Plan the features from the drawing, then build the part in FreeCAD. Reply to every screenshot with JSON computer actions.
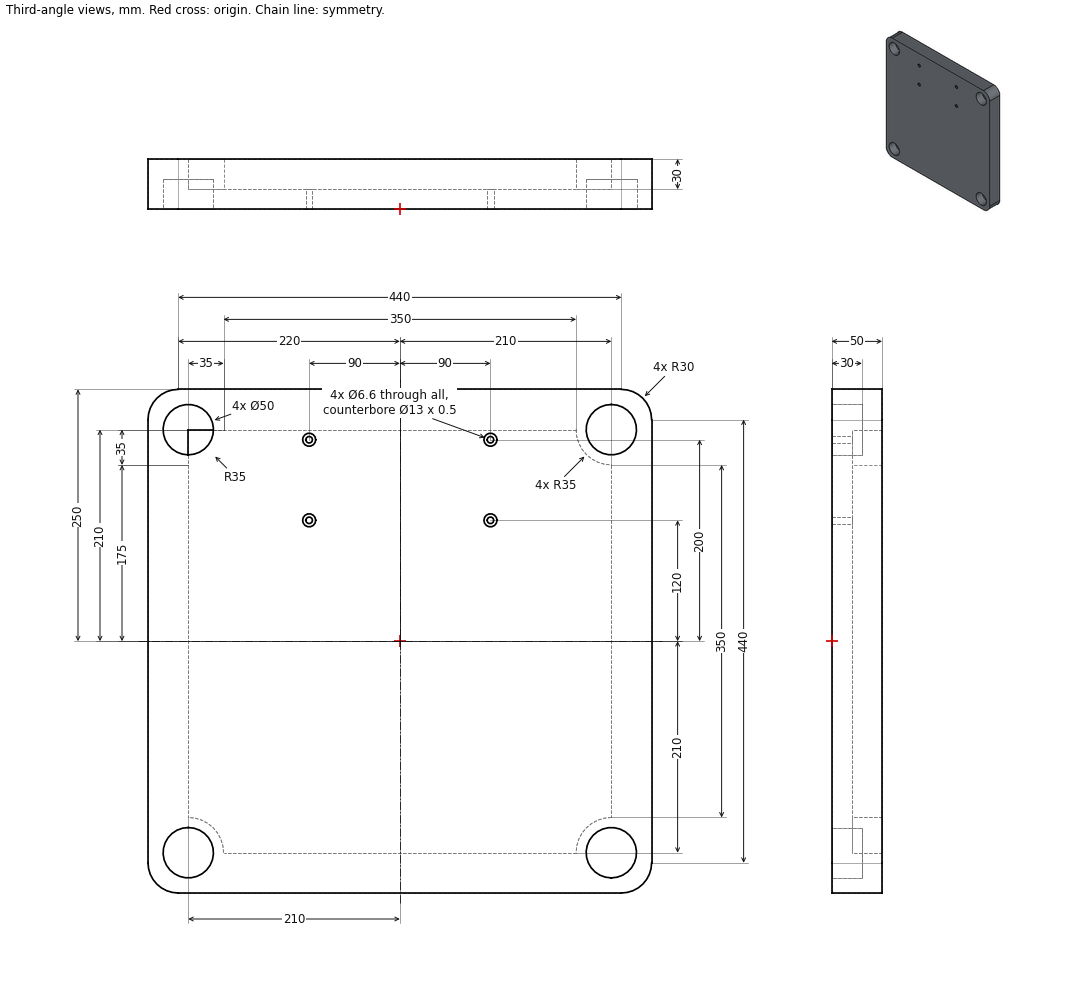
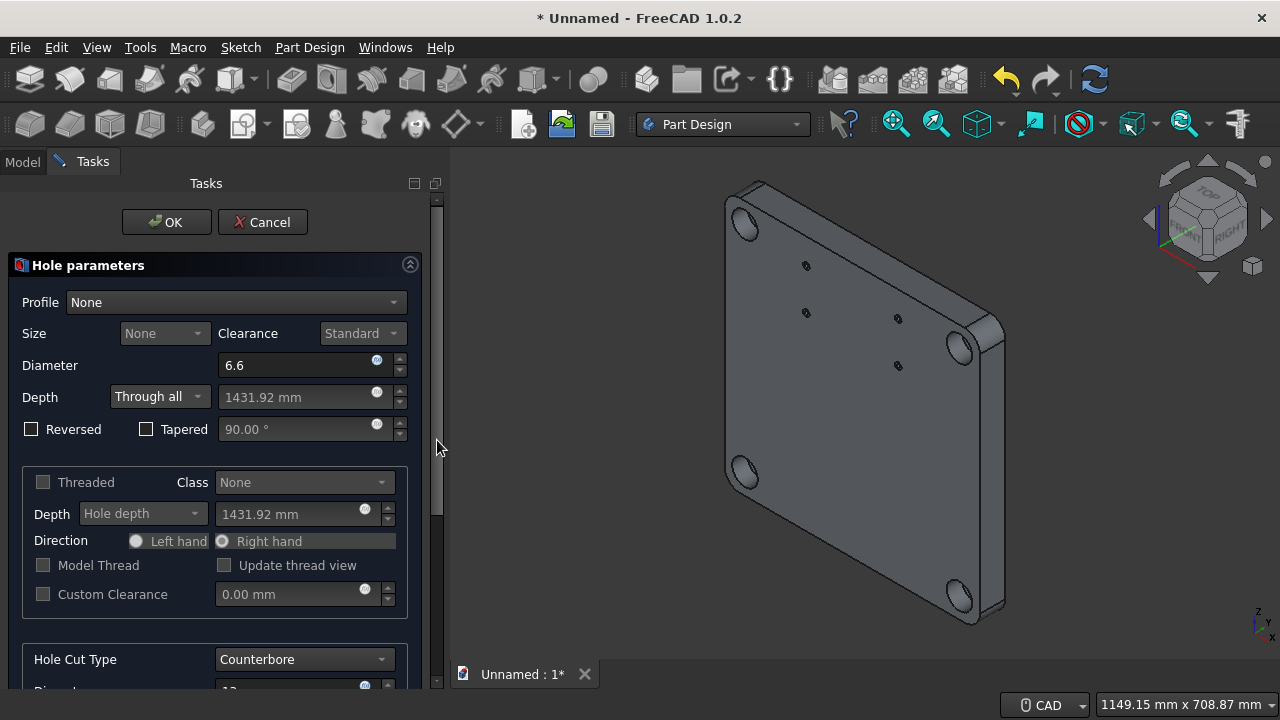
{"action": "left_click", "coordinate": [167, 222]}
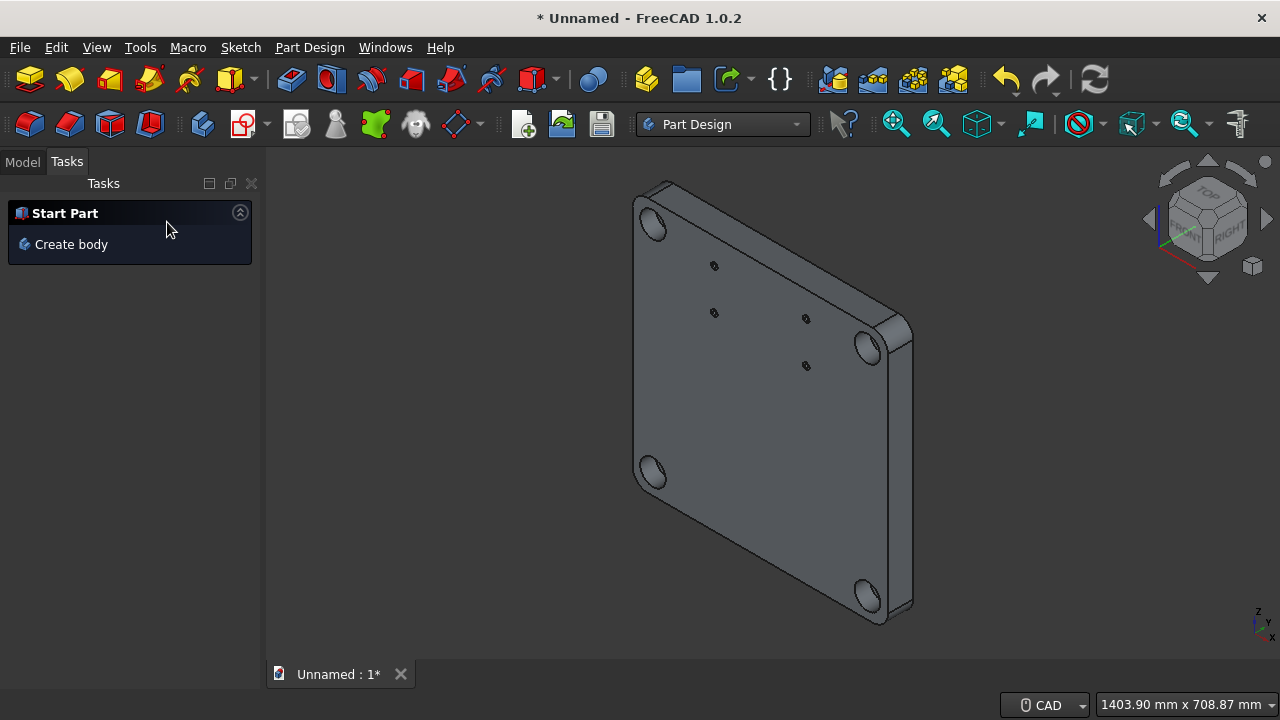
{"action": "key", "text": "4"}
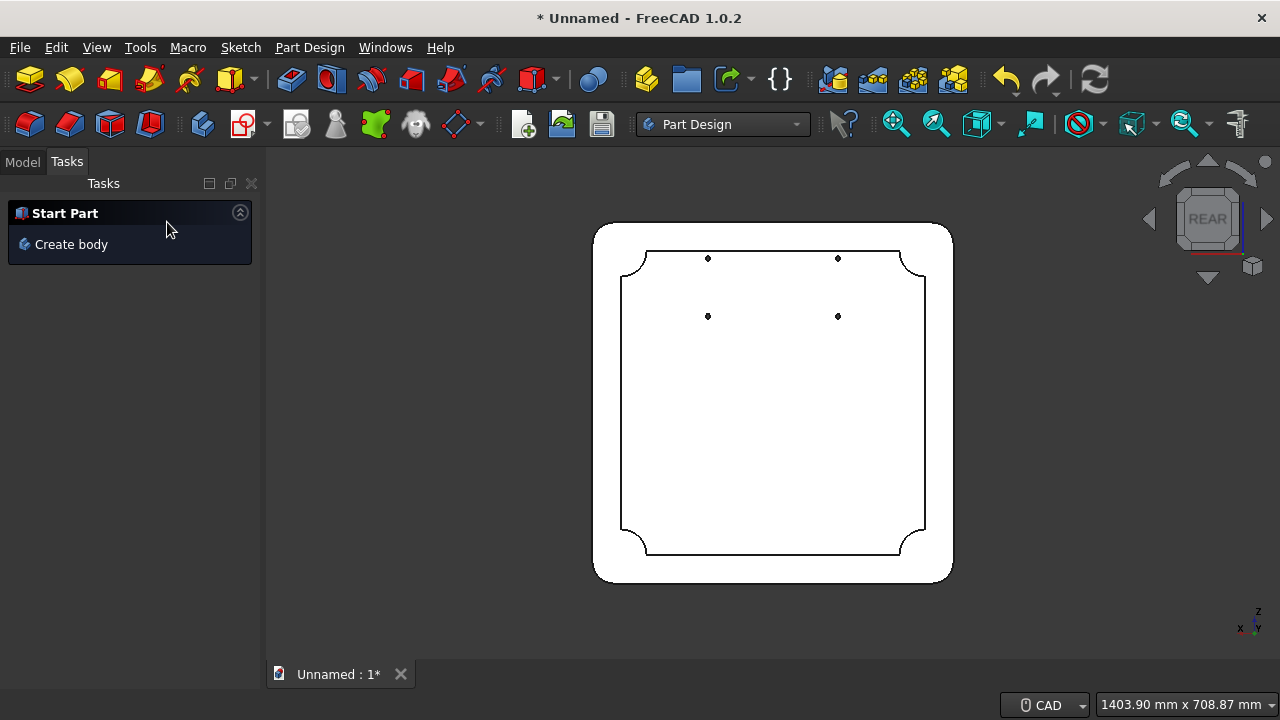
{"action": "left_click", "coordinate": [618, 247]}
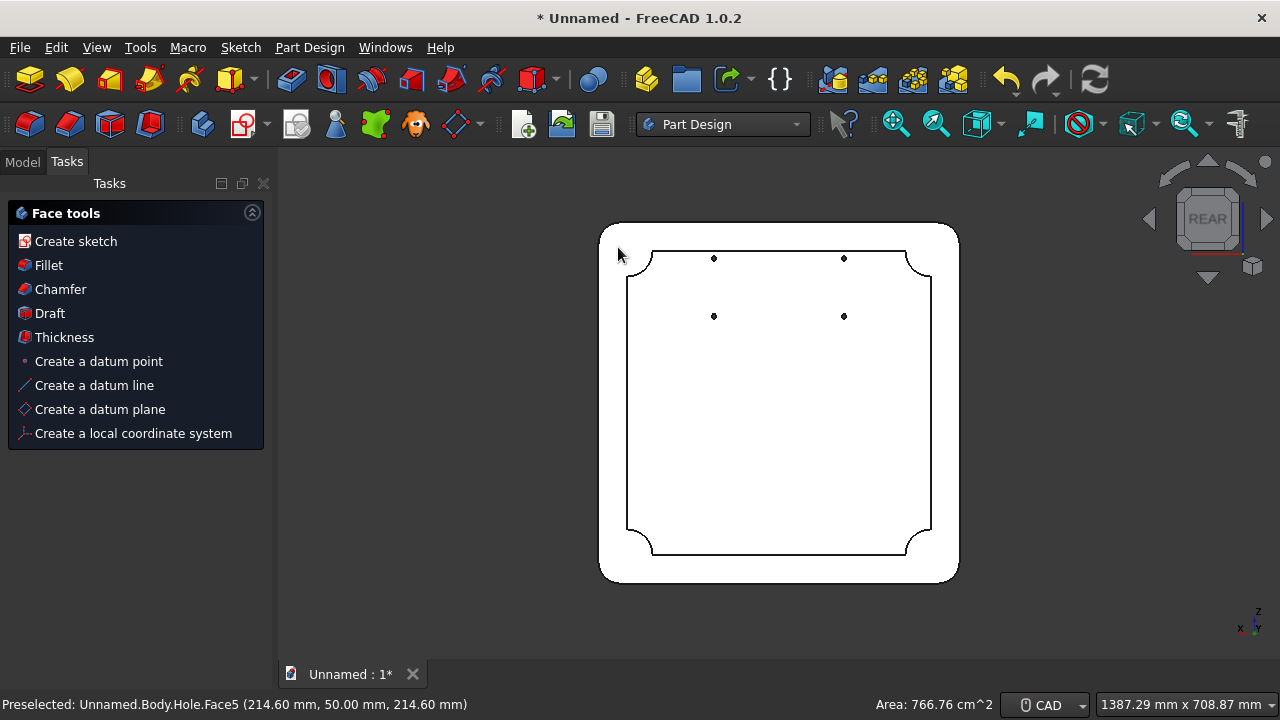
{"action": "left_click", "coordinate": [244, 124]}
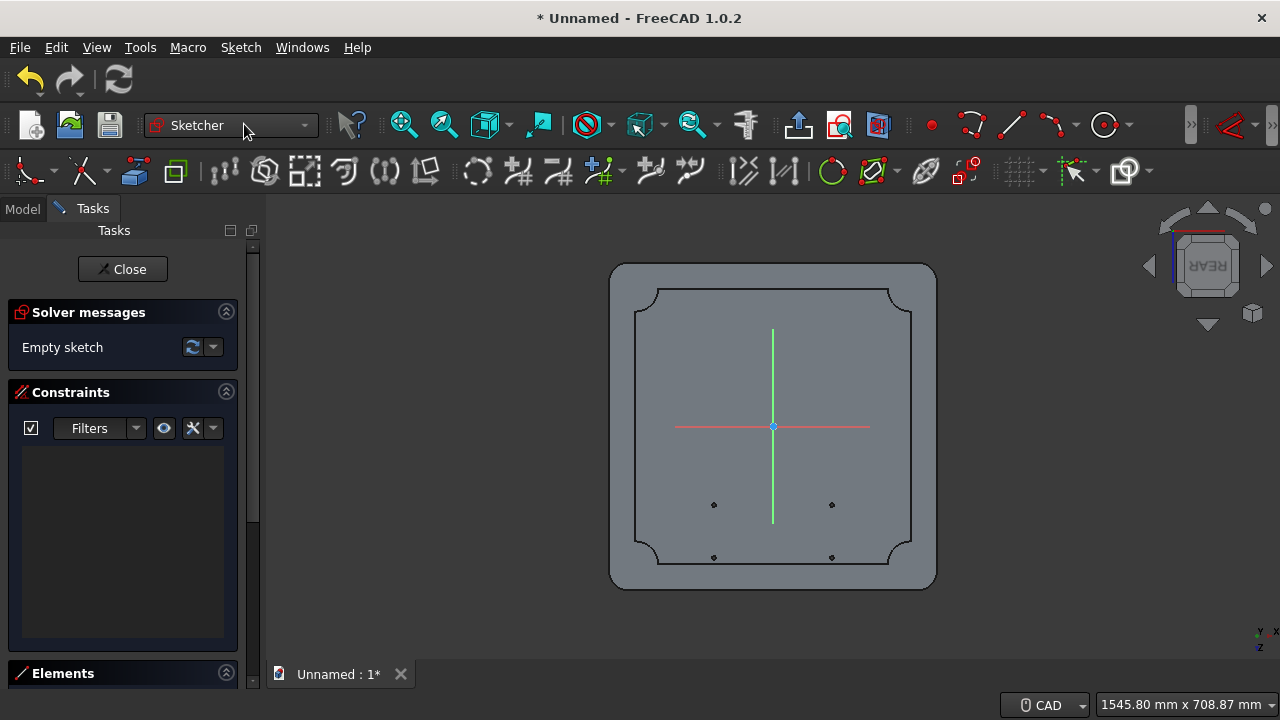
{"action": "scroll", "coordinate": [642, 563], "scroll_direction": "up", "scroll_amount": 13}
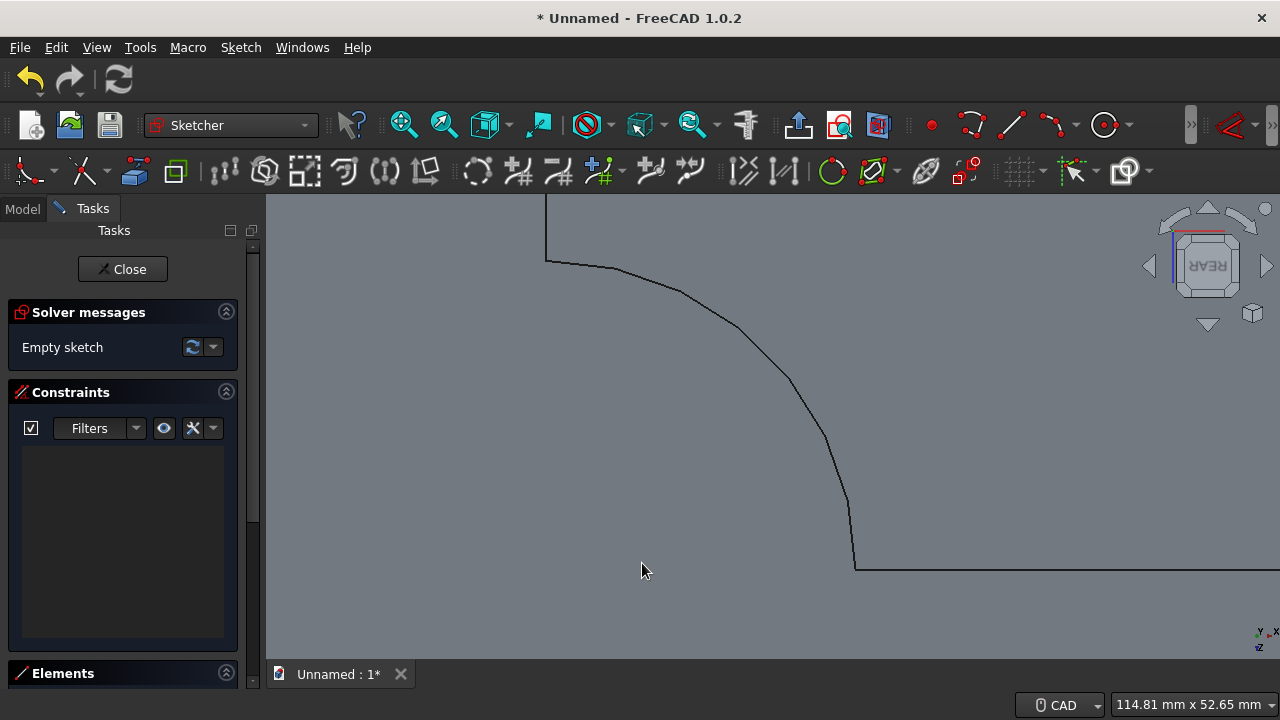
{"action": "left_click", "coordinate": [972, 126]}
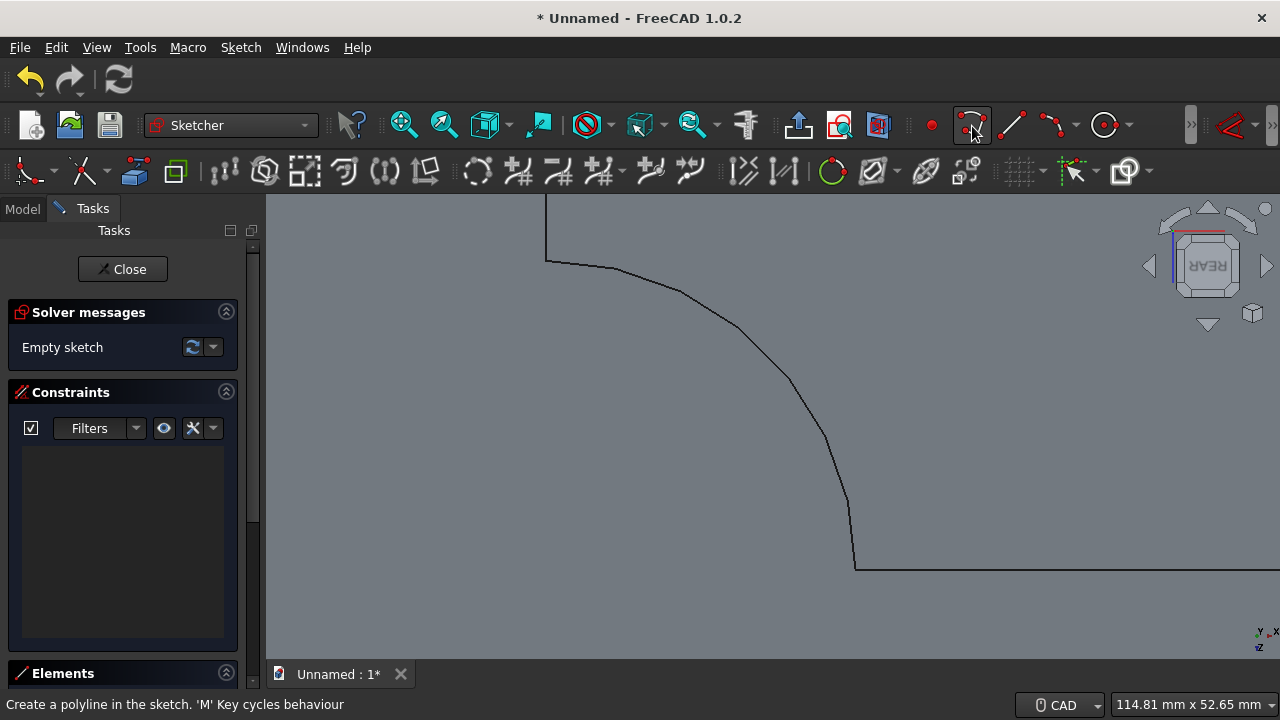
{"action": "left_click", "coordinate": [546, 261]}
{"action": "left_click", "coordinate": [546, 570]}
{"action": "left_click", "coordinate": [856, 570]}
{"action": "right_click", "coordinate": [856, 570]}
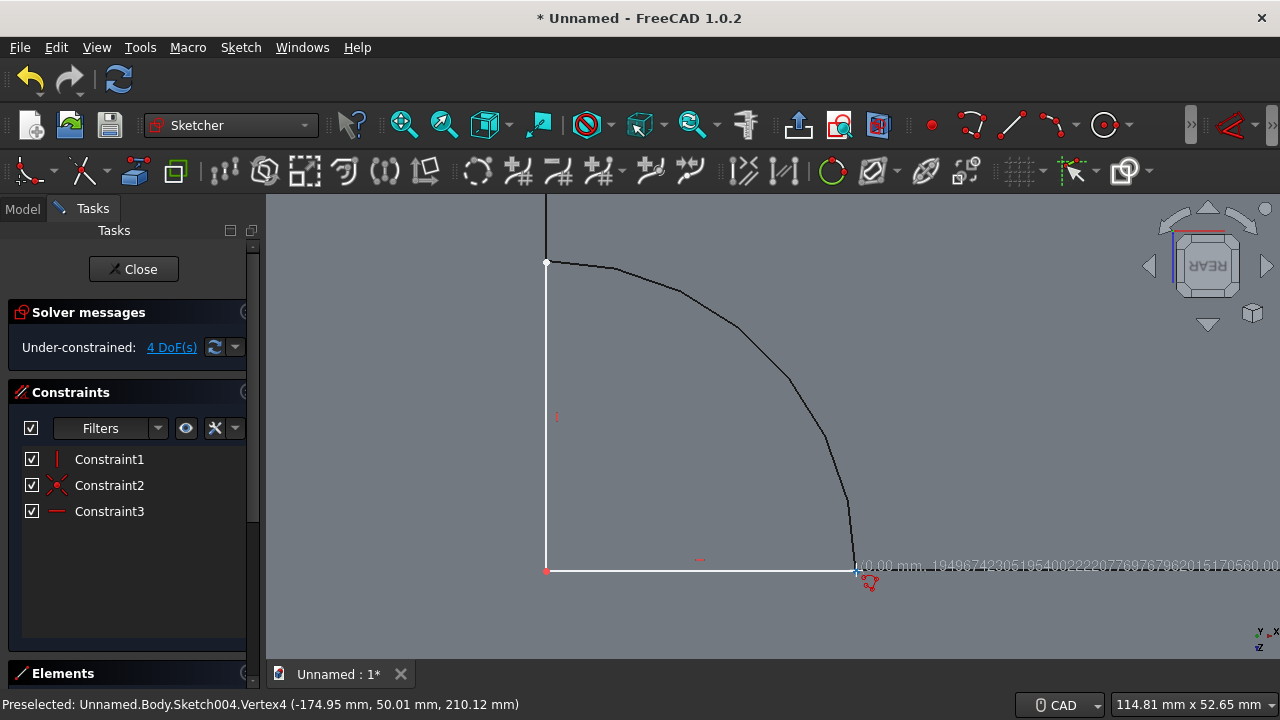
{"action": "key", "text": "g 3 a"}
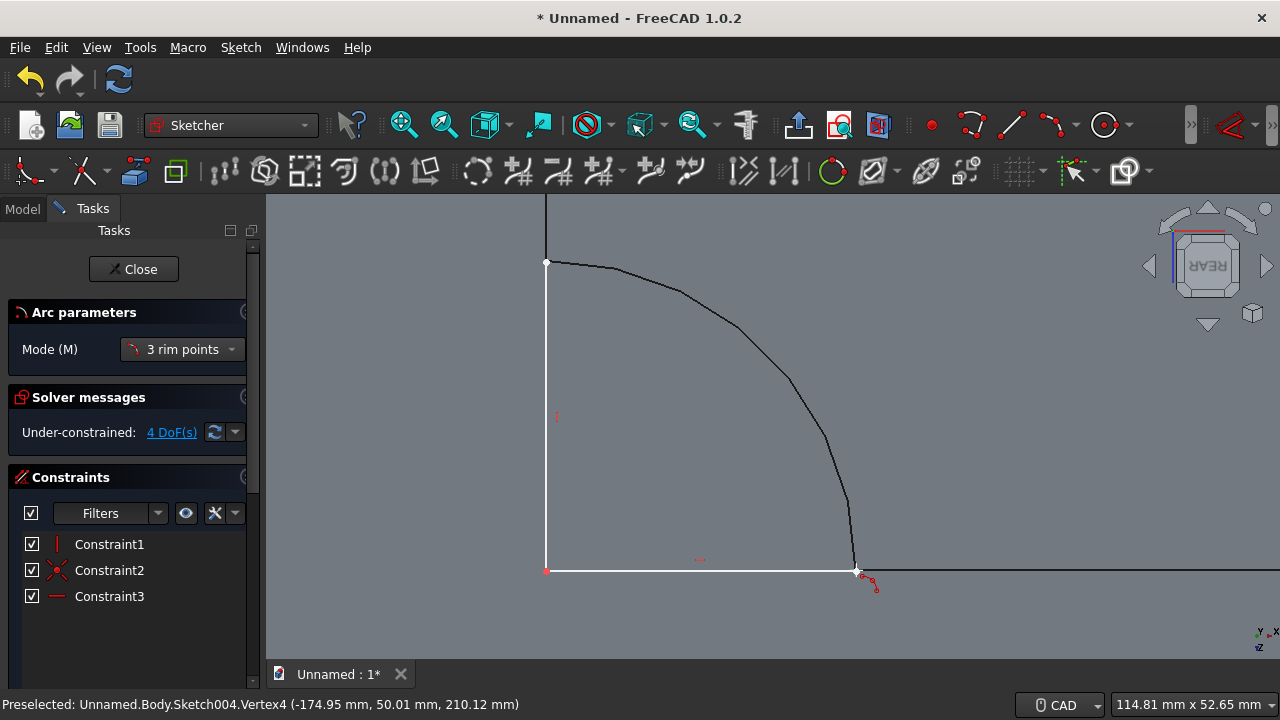
{"action": "left_click", "coordinate": [856, 571]}
{"action": "left_click", "coordinate": [546, 262]}
{"action": "left_click", "coordinate": [765, 351]}
{"action": "key", "text": "Escape"}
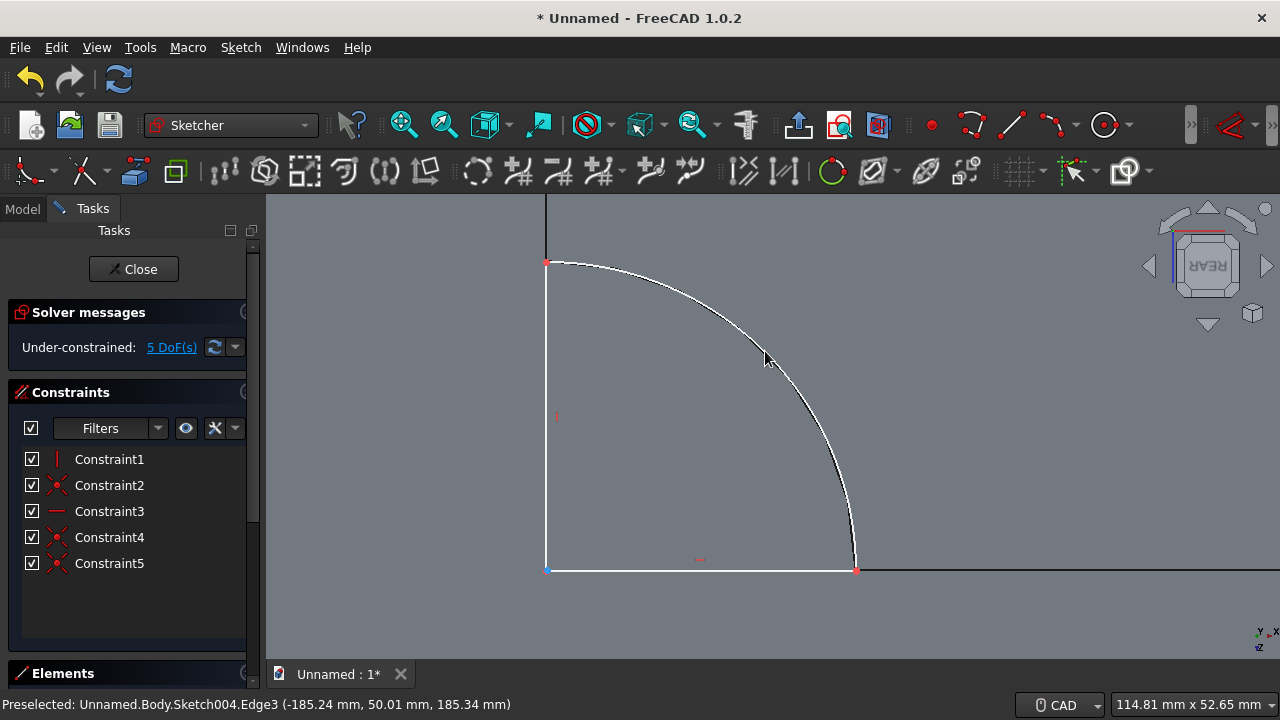
{"action": "left_click", "coordinate": [1230, 126]}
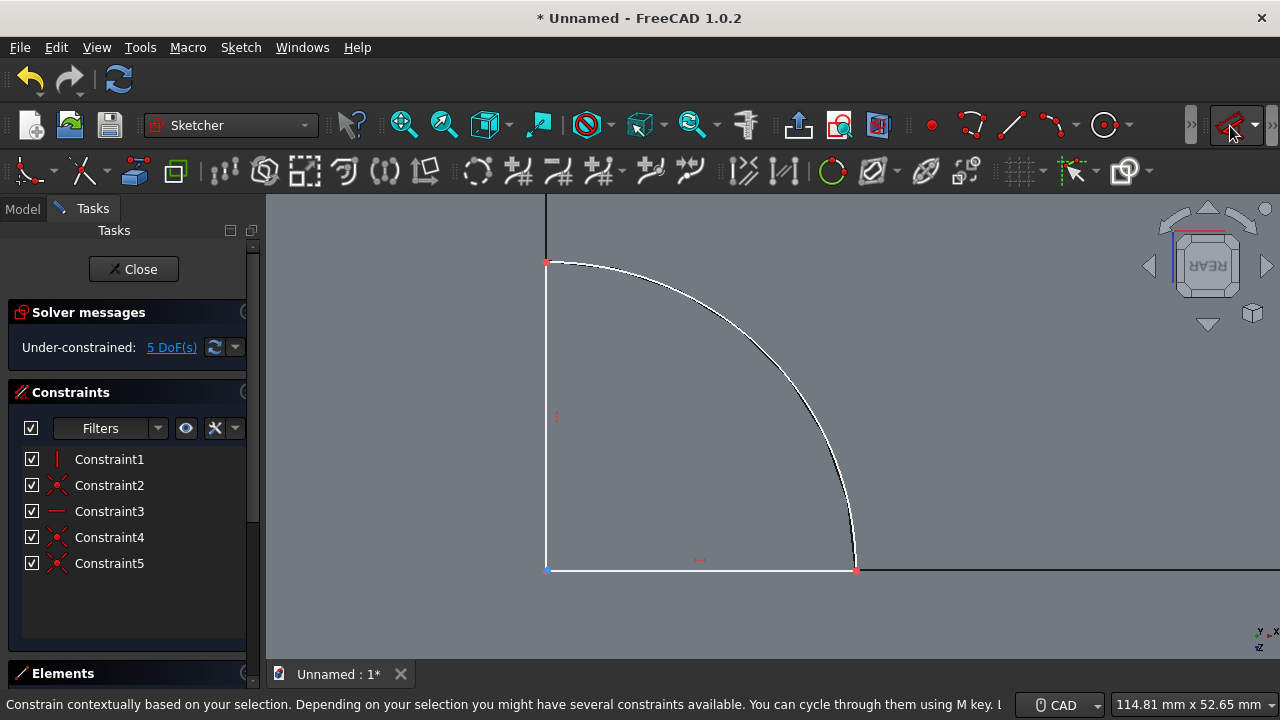
{"action": "left_click", "coordinate": [822, 430]}
{"action": "left_click", "coordinate": [850, 415]}